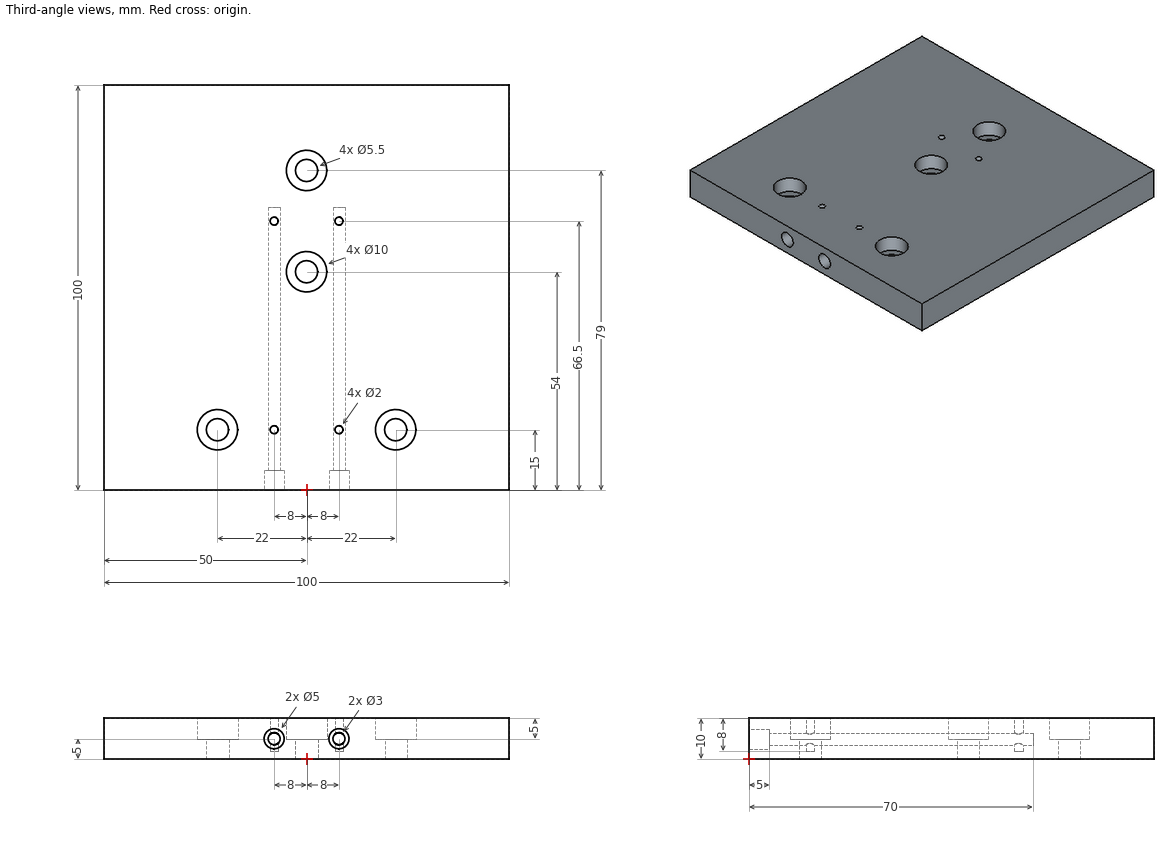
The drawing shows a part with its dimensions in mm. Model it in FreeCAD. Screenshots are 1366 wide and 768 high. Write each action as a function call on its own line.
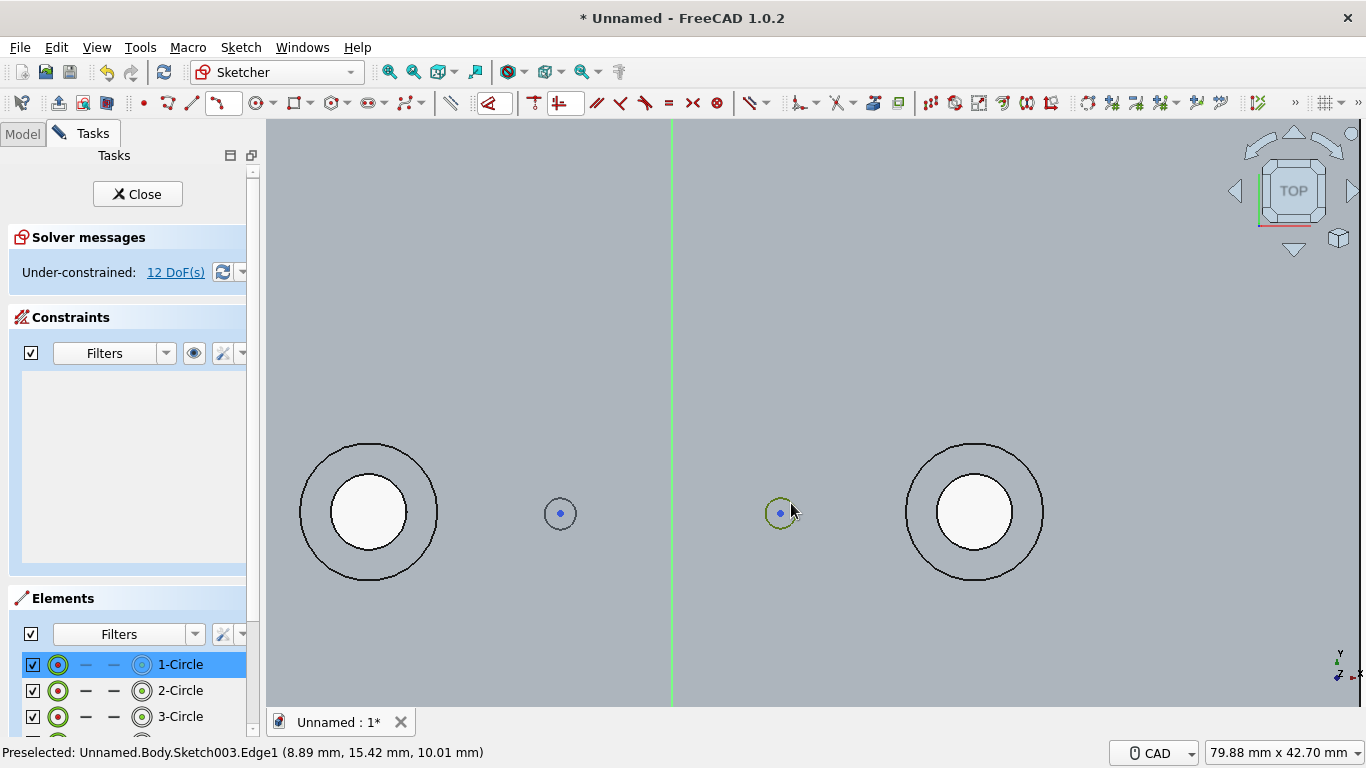
click(571, 503)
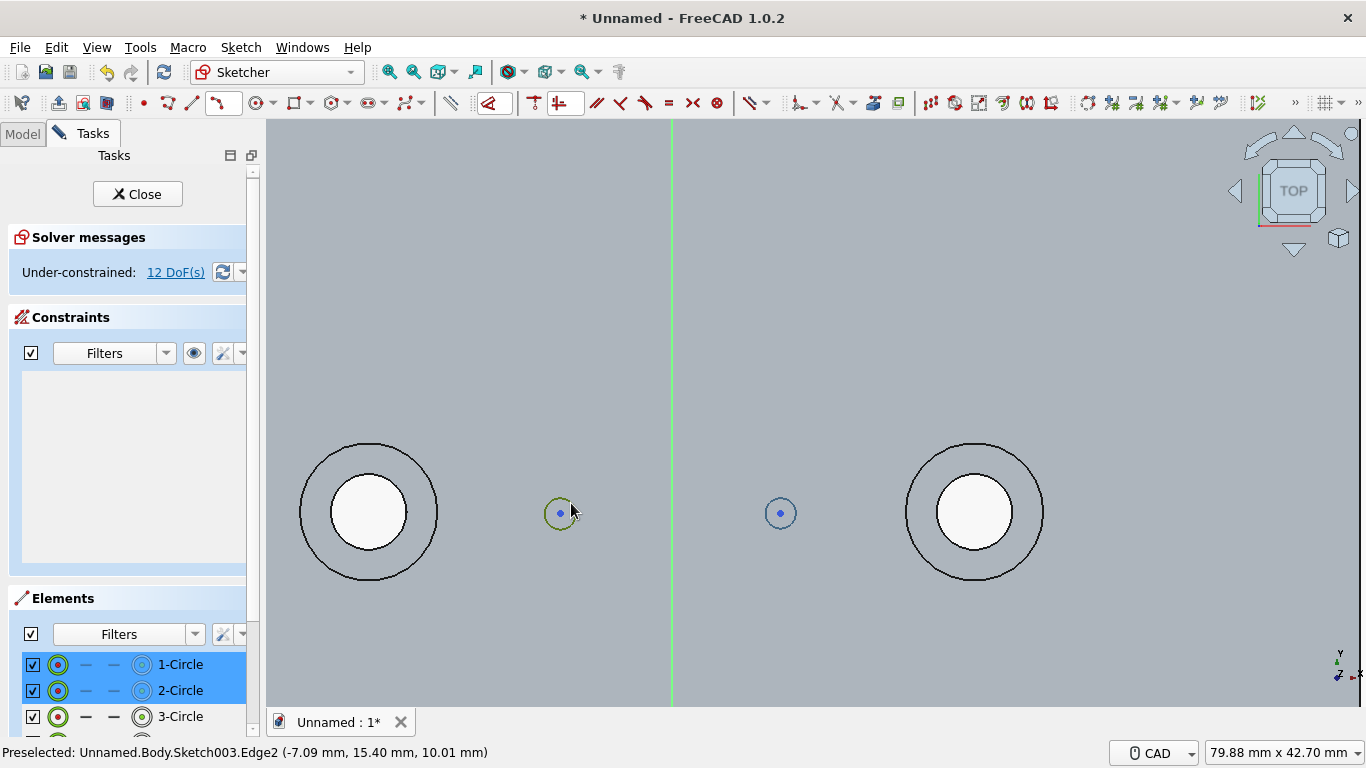
scroll(792, 506, down, 5)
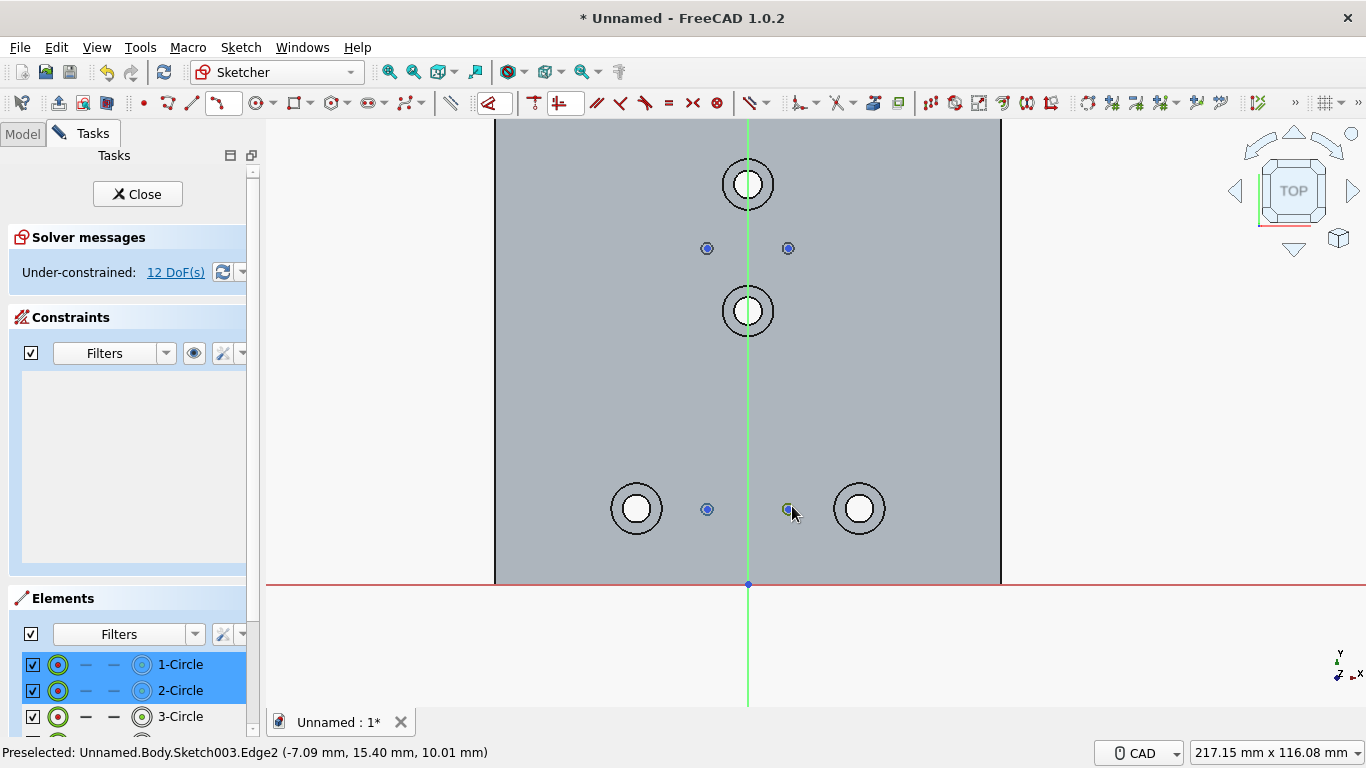
scroll(792, 244, up, 5)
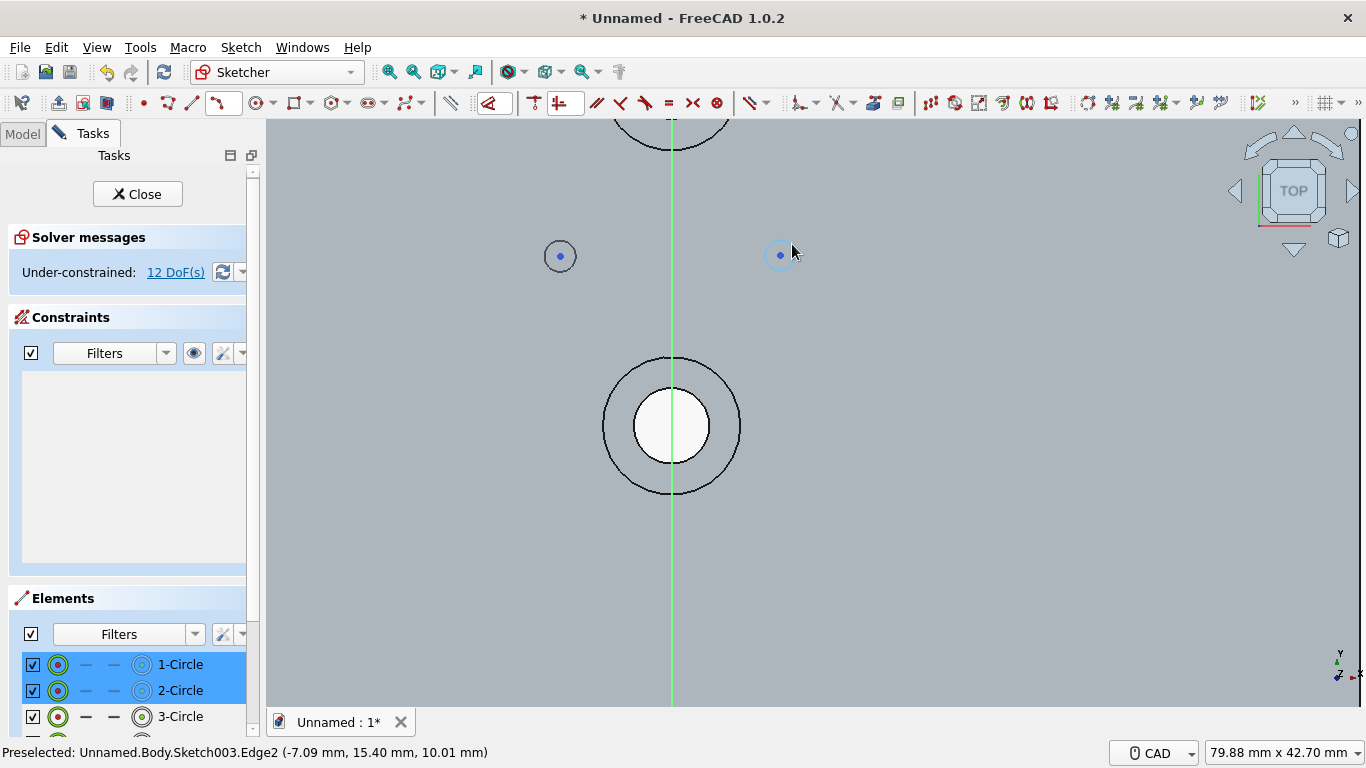
click(791, 245)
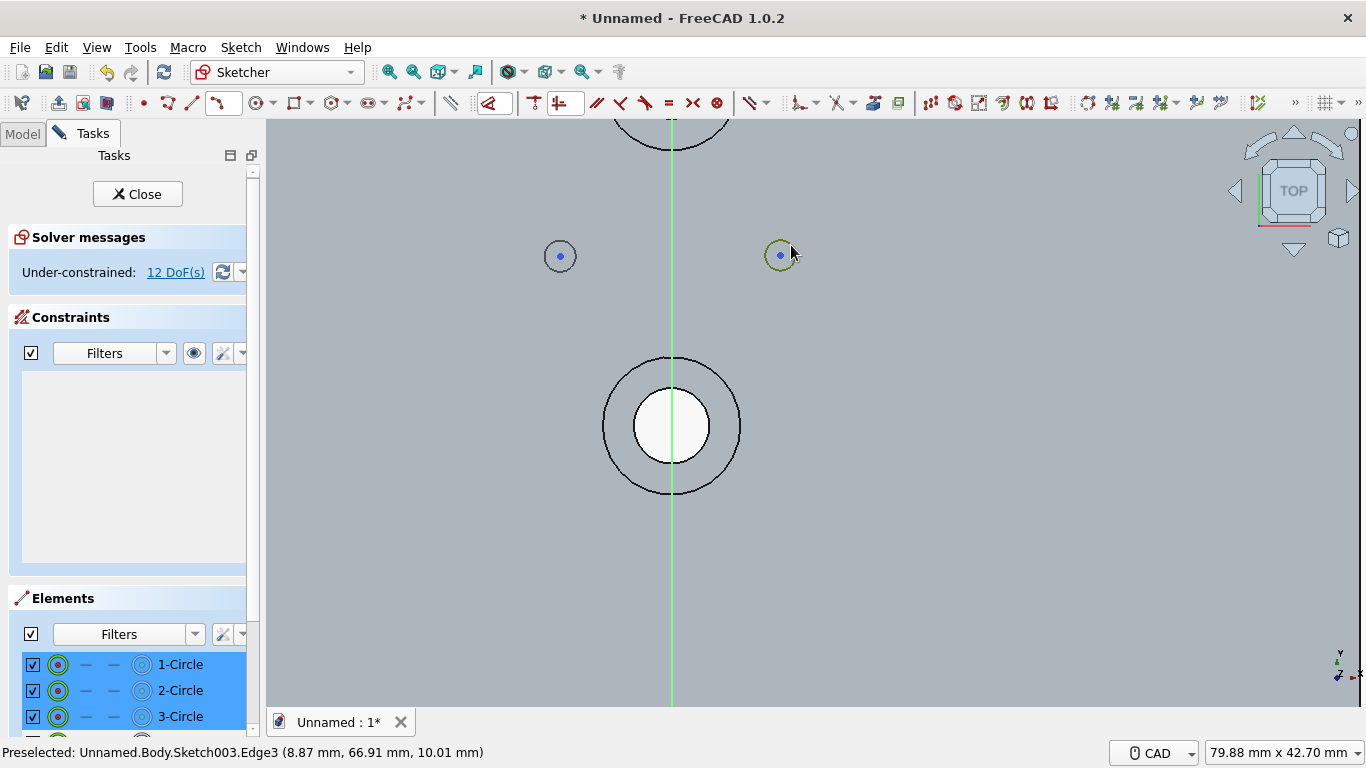
click(571, 245)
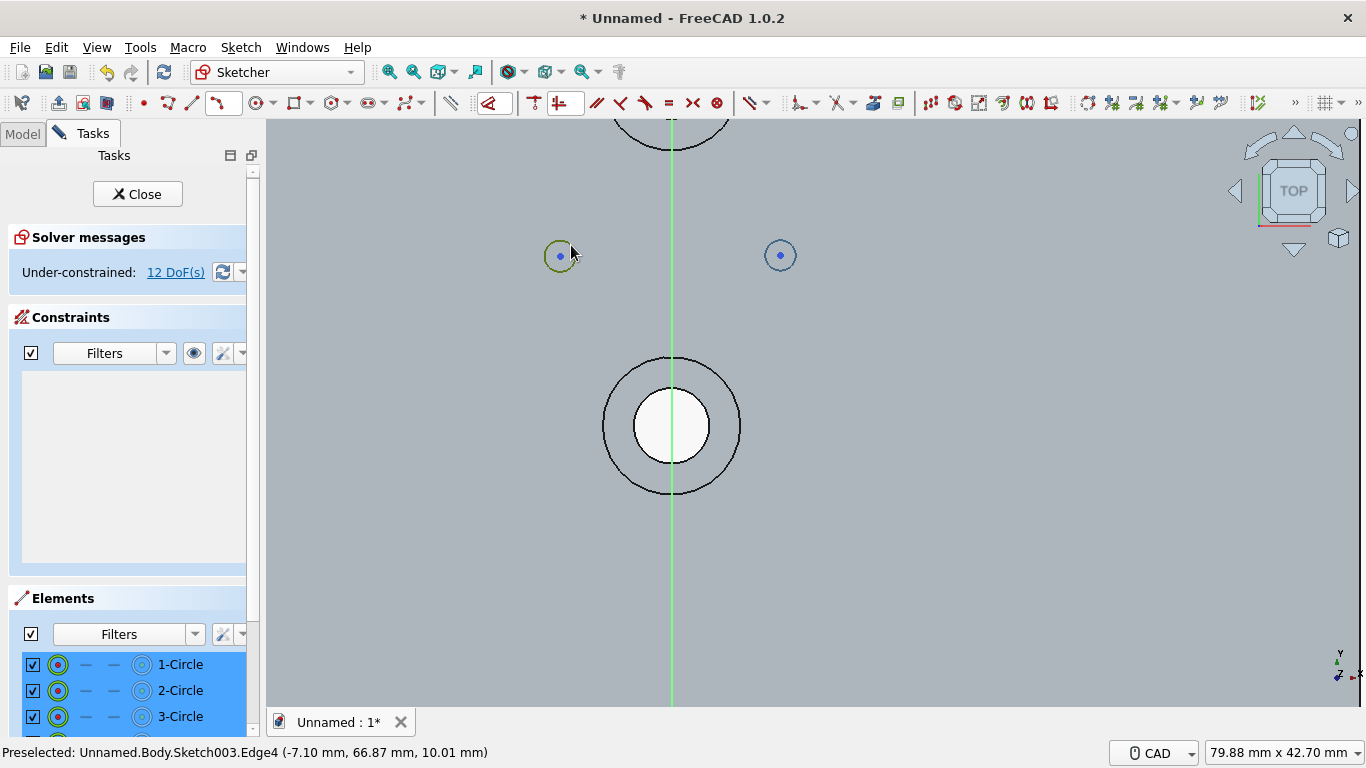
click(670, 104)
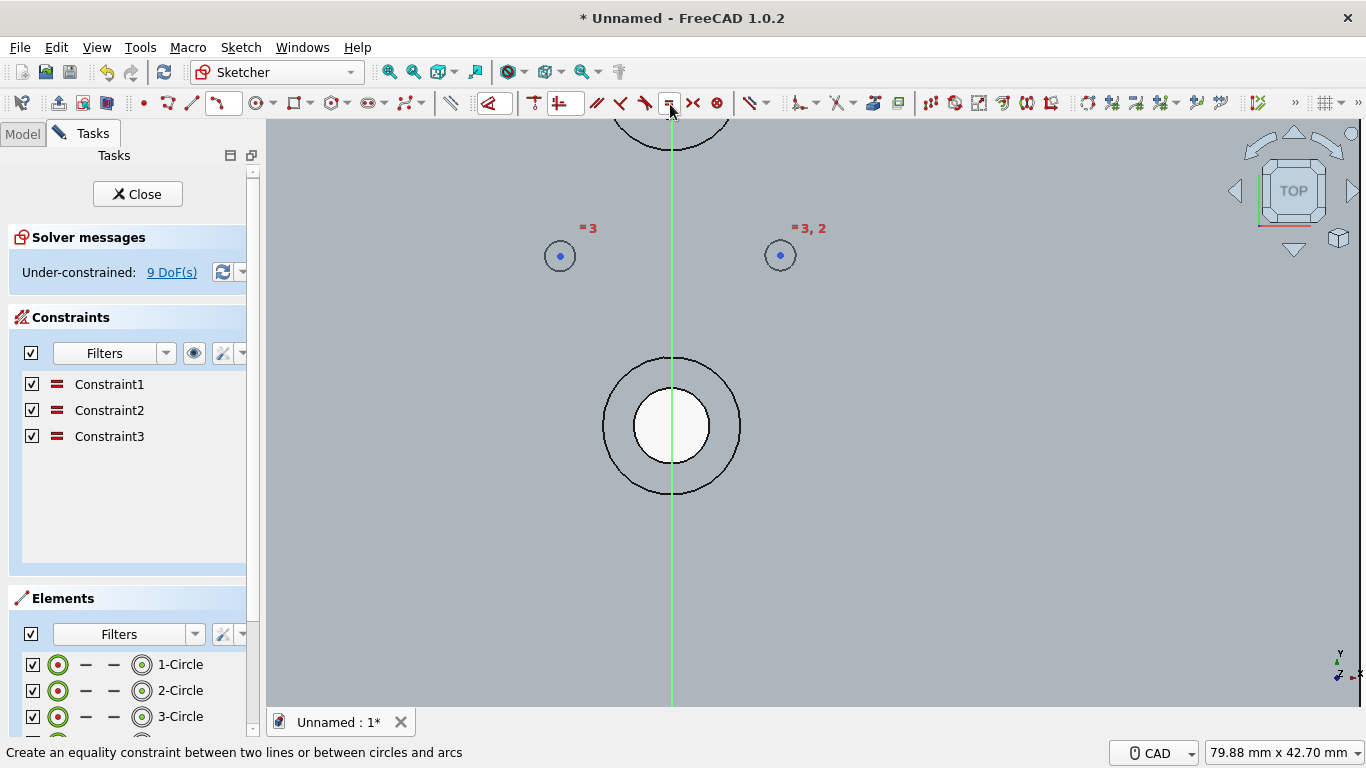
scroll(792, 243, down, 5)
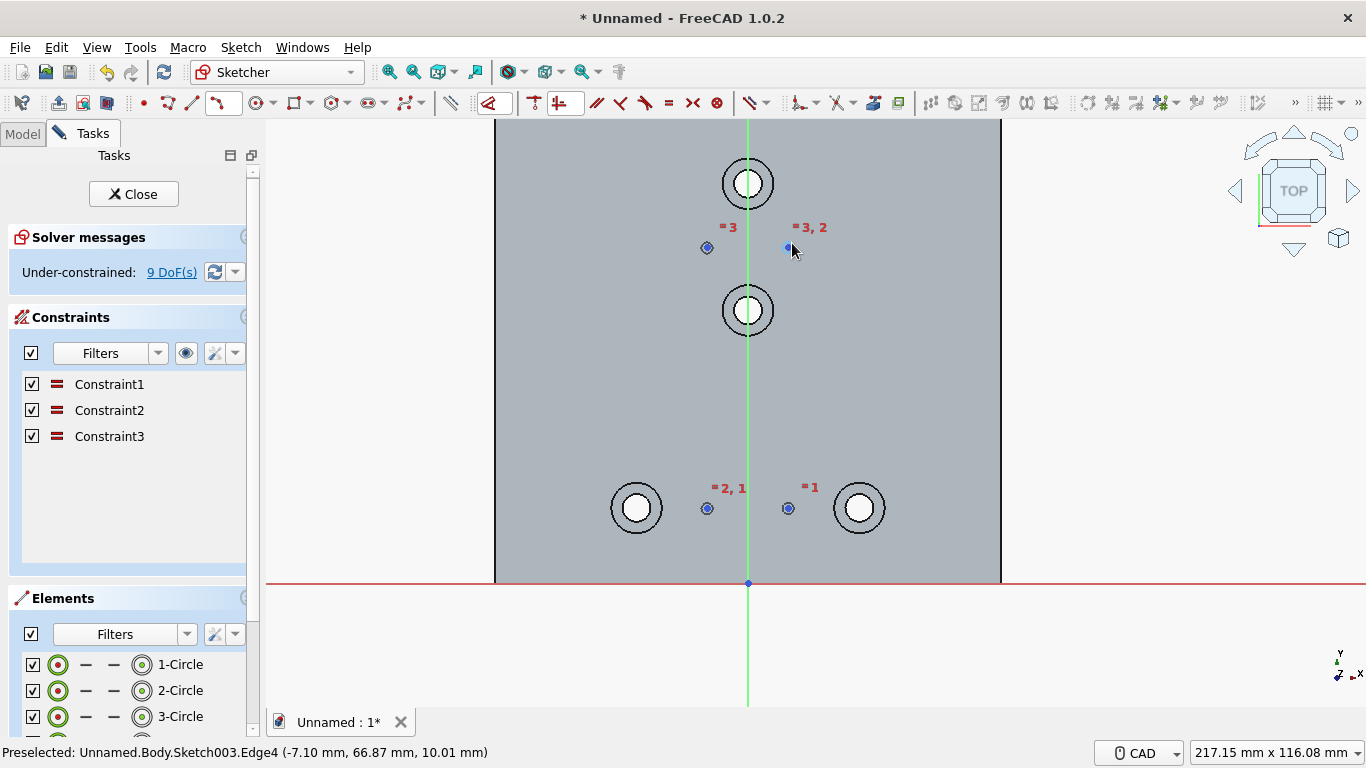
scroll(792, 505, up, 7)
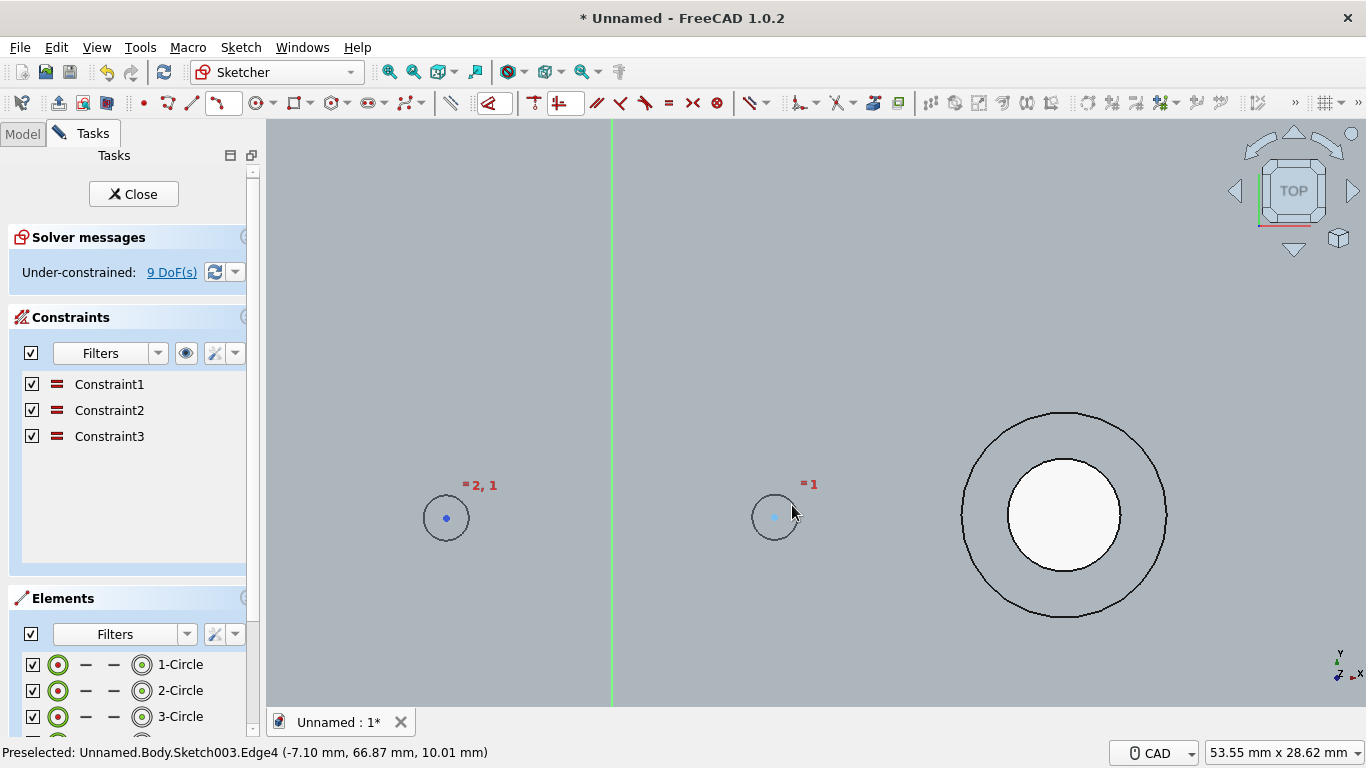
click(791, 501)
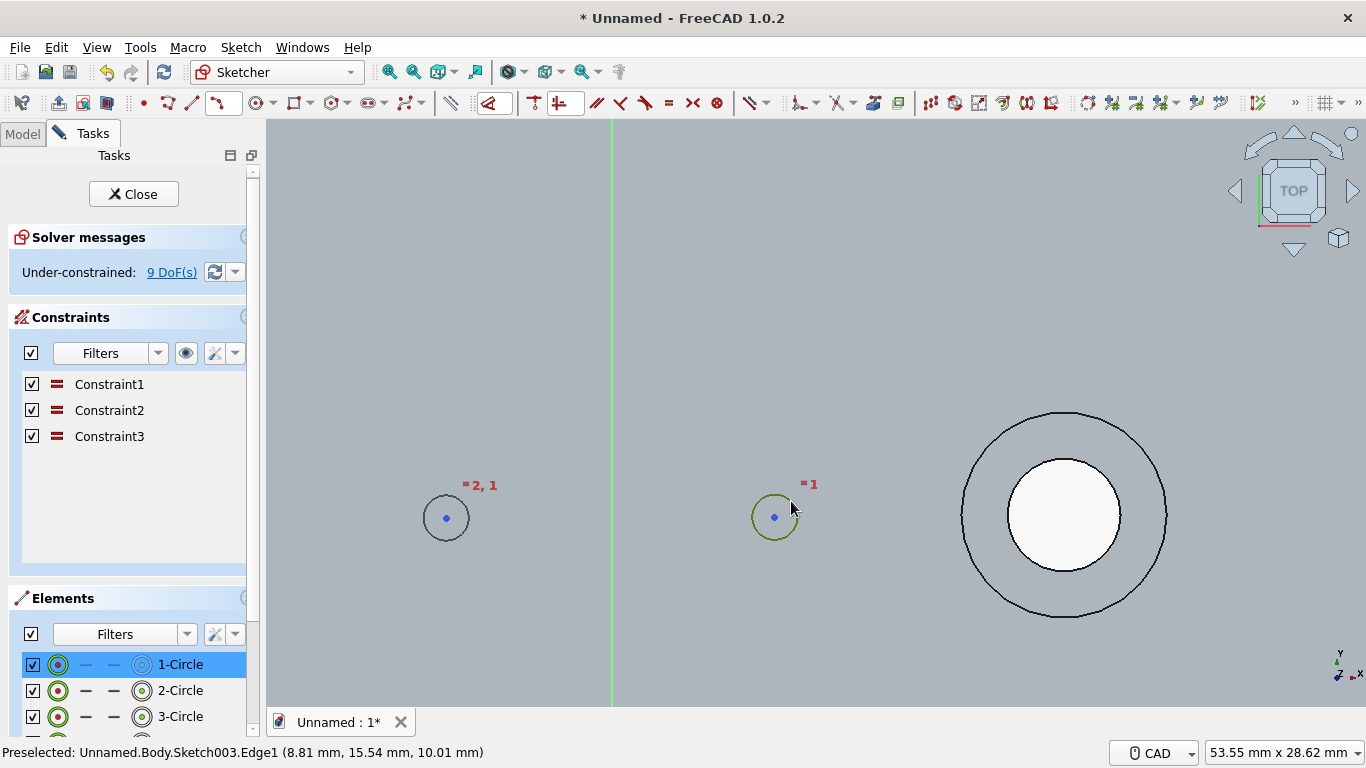
key(k)
key(o)